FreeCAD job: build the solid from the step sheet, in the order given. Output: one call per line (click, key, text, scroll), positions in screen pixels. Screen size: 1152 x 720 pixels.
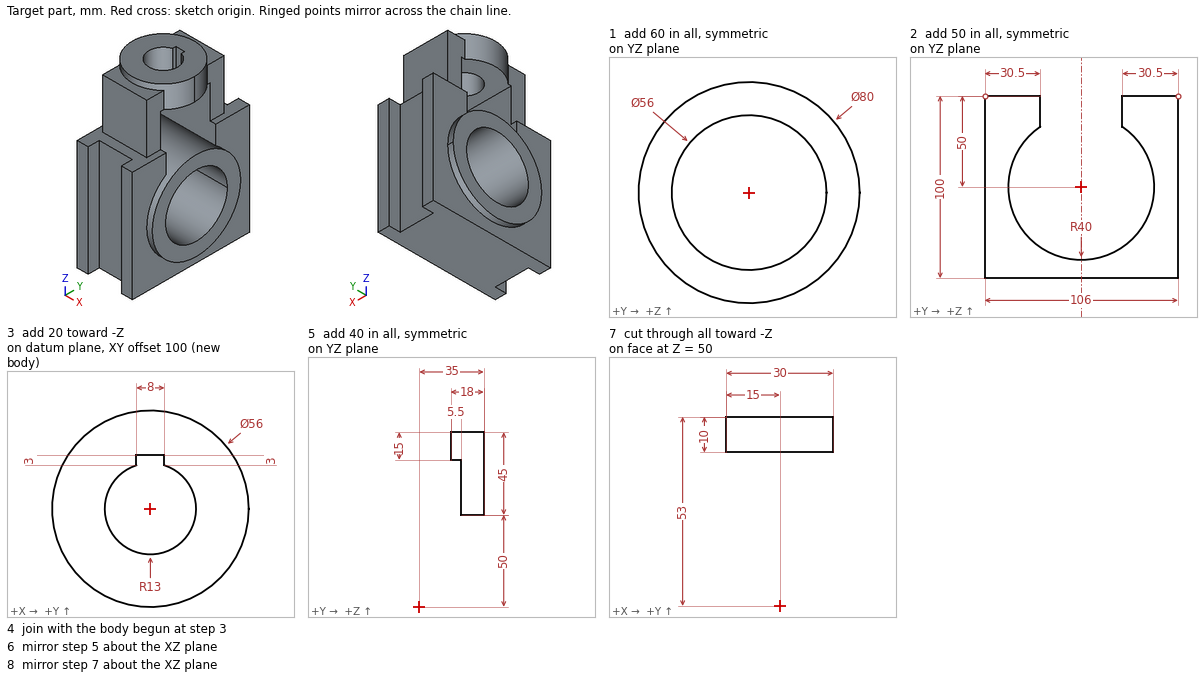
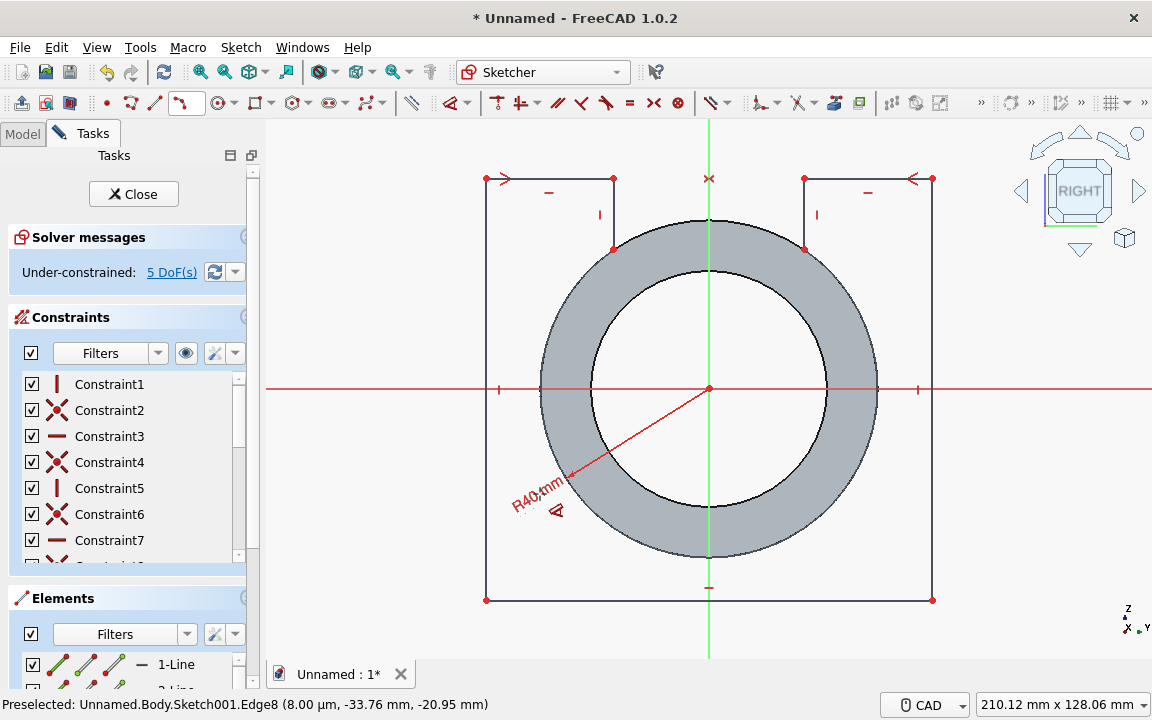
click(486, 306)
click(452, 293)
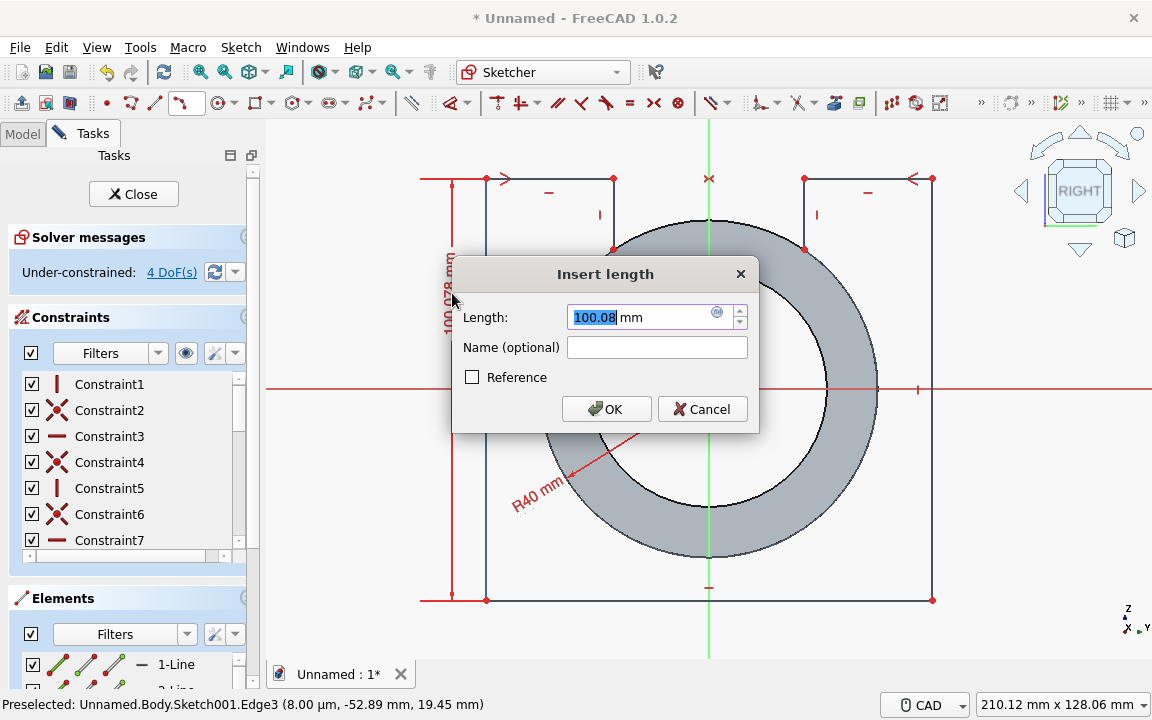
text(100)
key(Return)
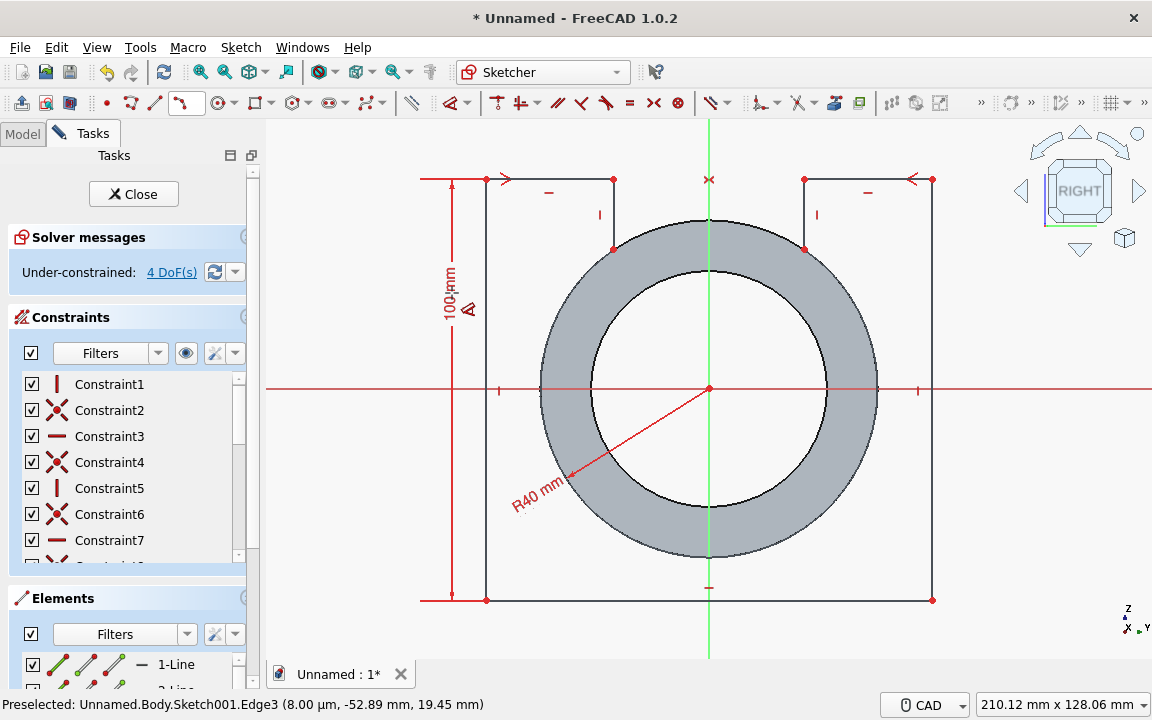
click(620, 601)
click(606, 567)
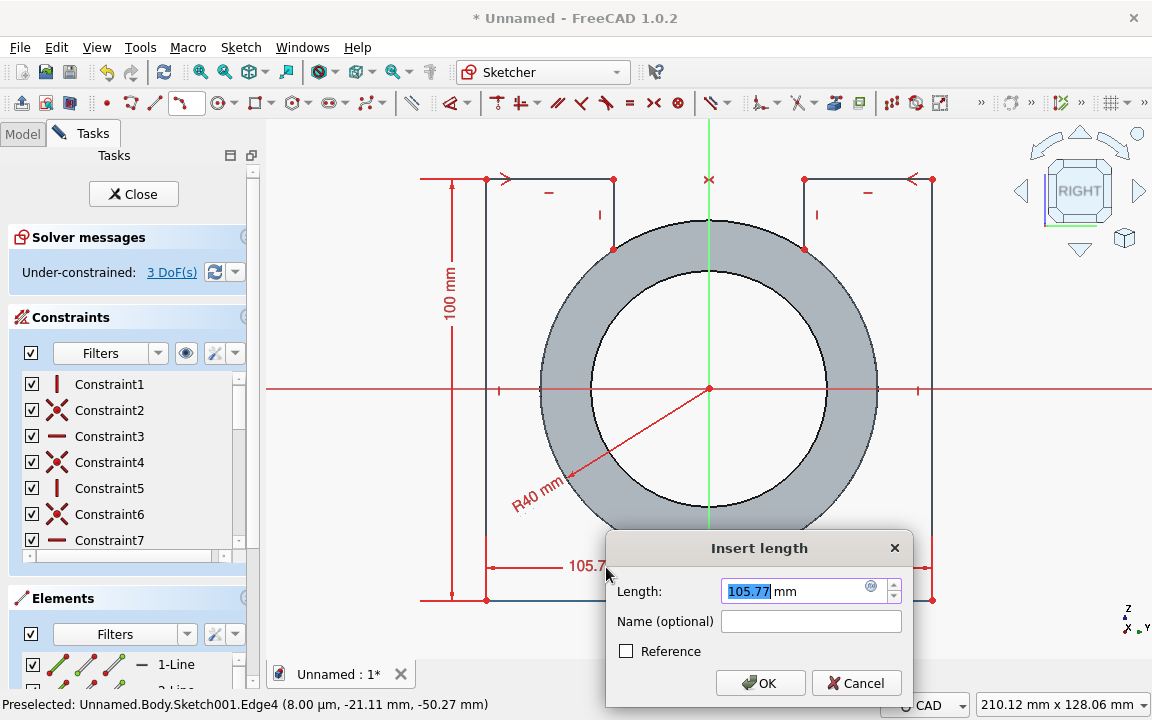
text(106)
key(Return)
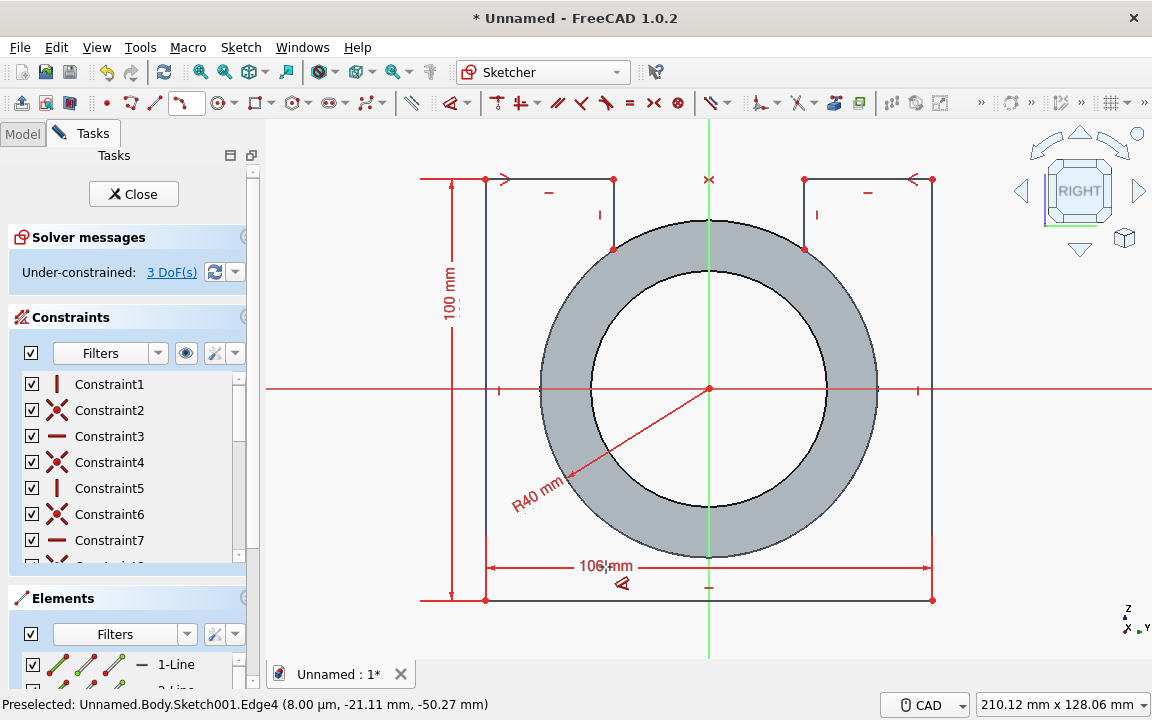
click(614, 179)
click(580, 236)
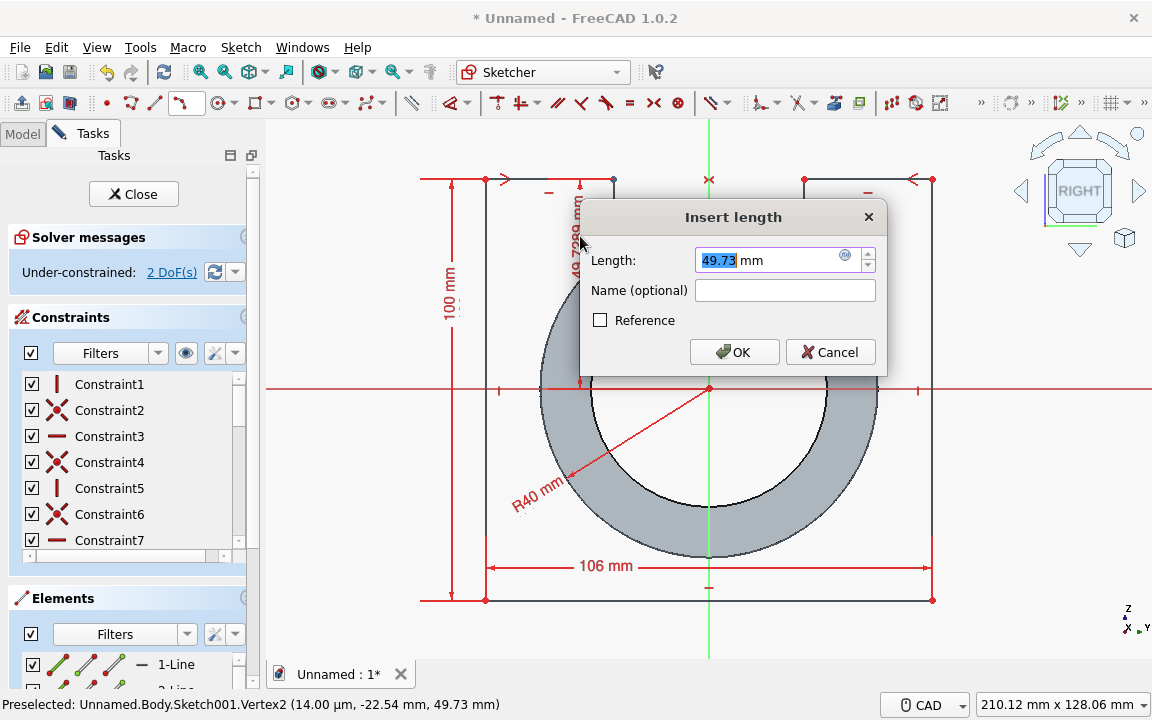
text(50)
key(Return)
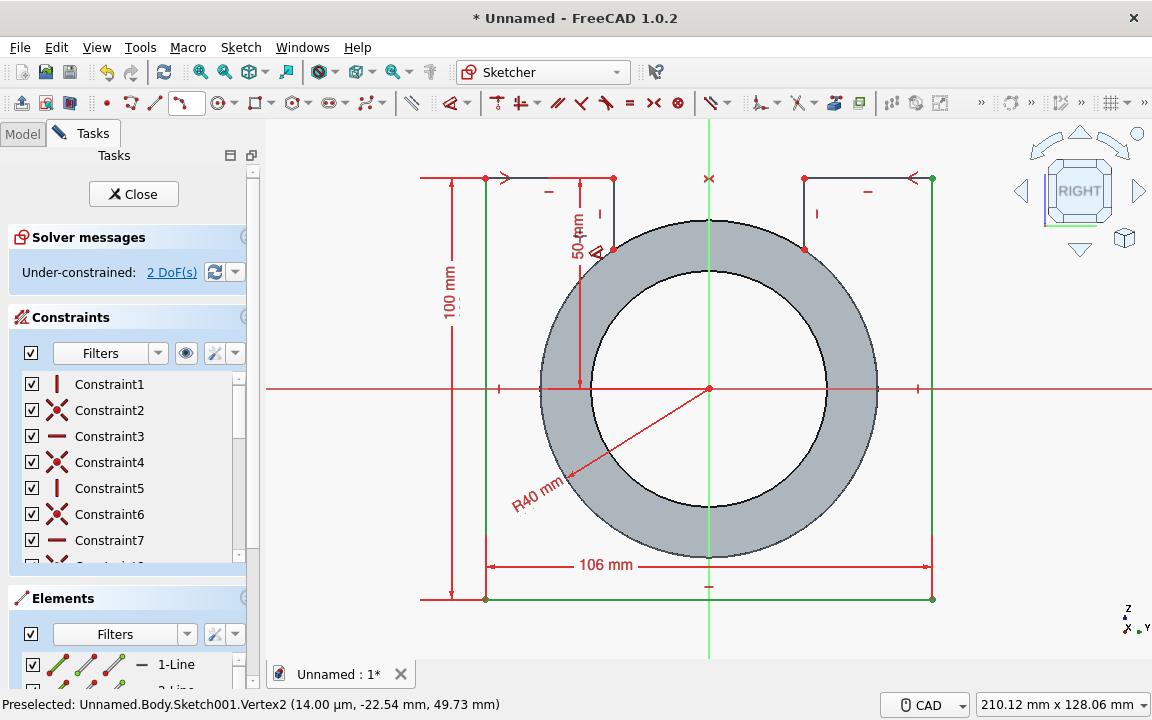
click(575, 178)
click(550, 212)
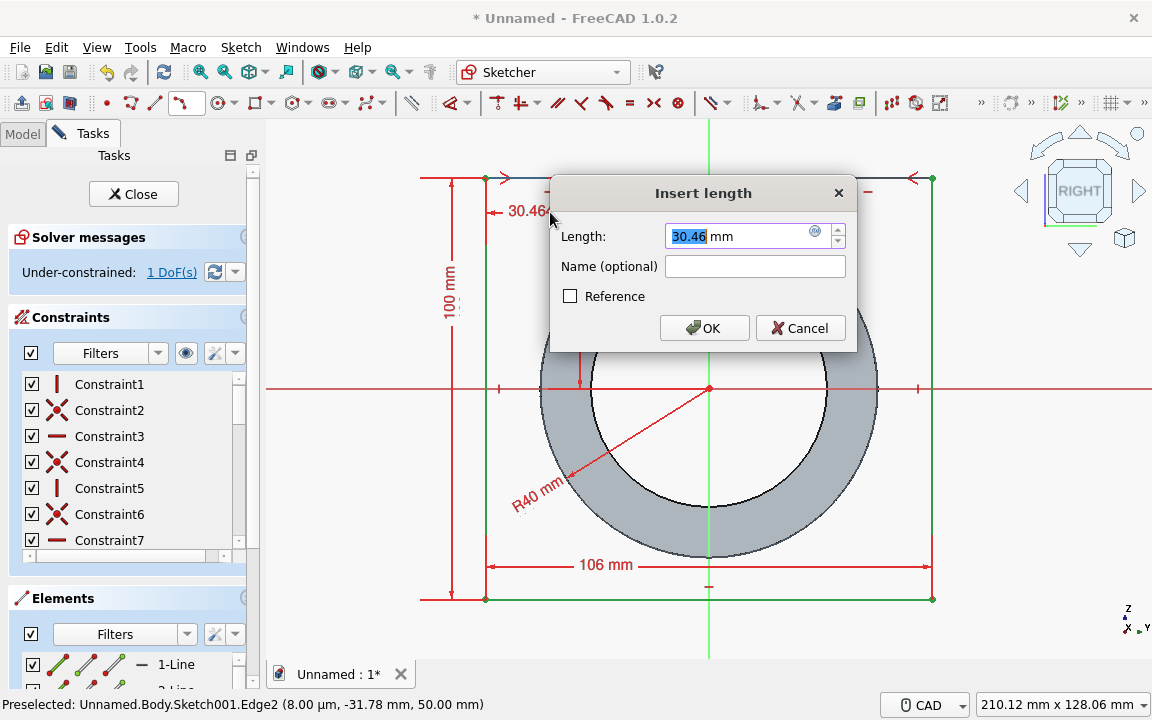
text(30.5)
key(Return)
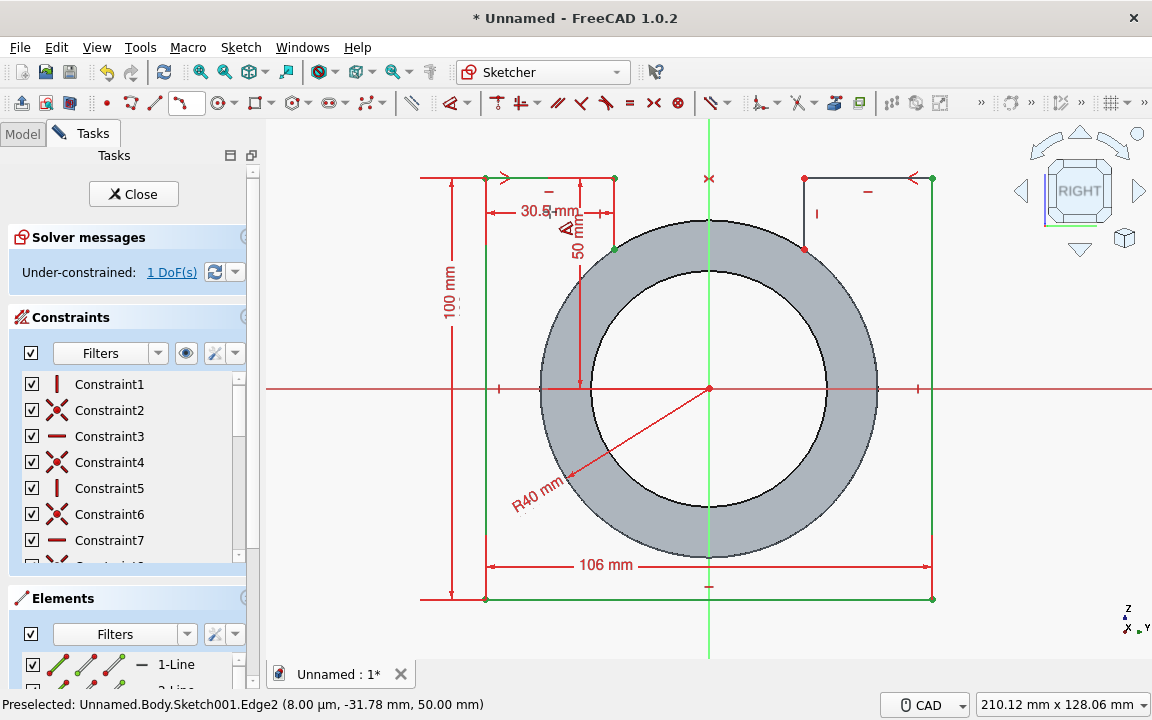
click(894, 178)
click(868, 212)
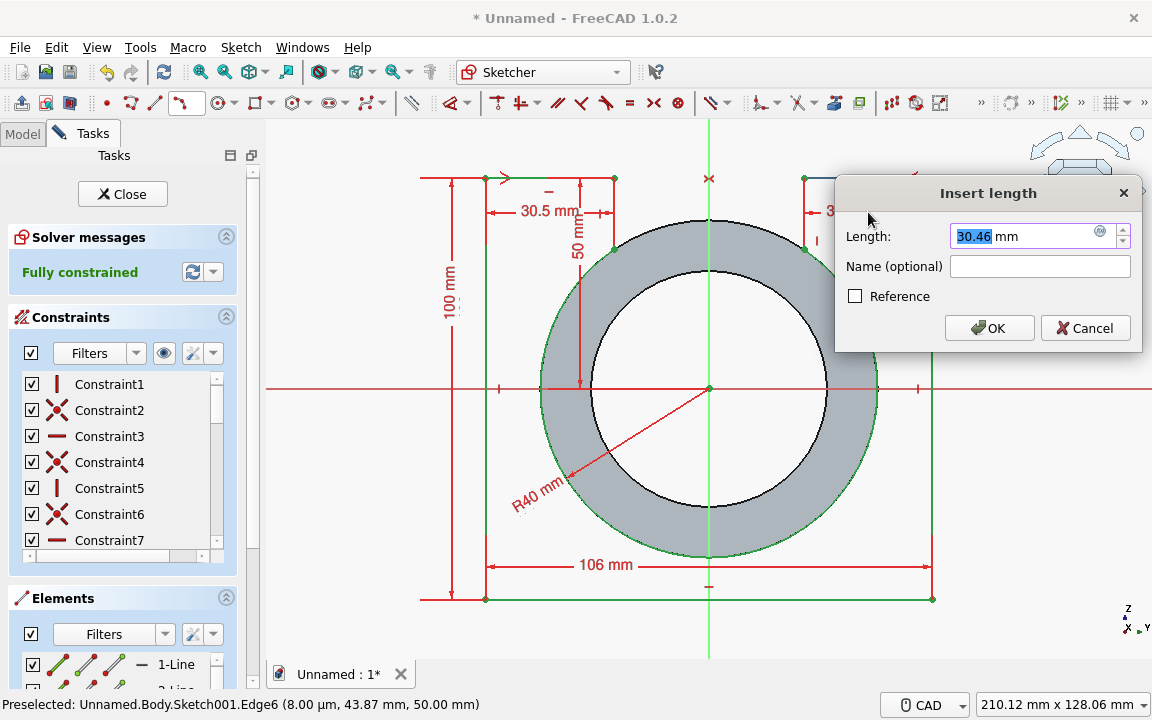
text(30.5)
key(Return)
key(Escape)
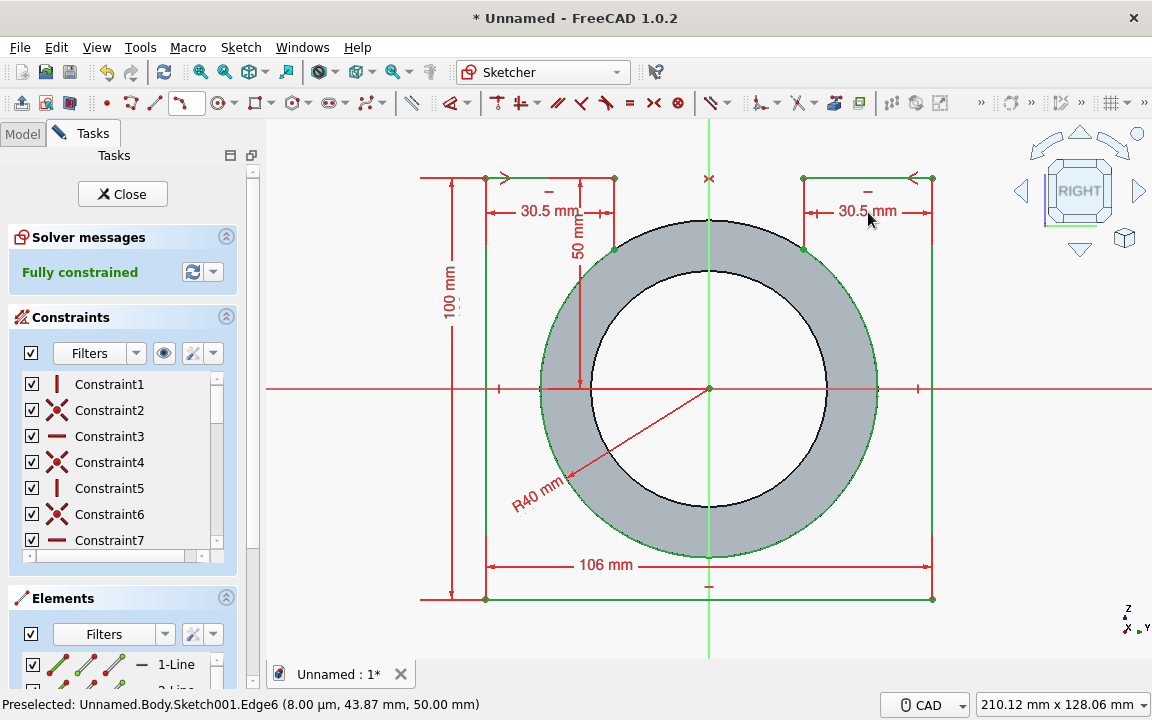
click(123, 194)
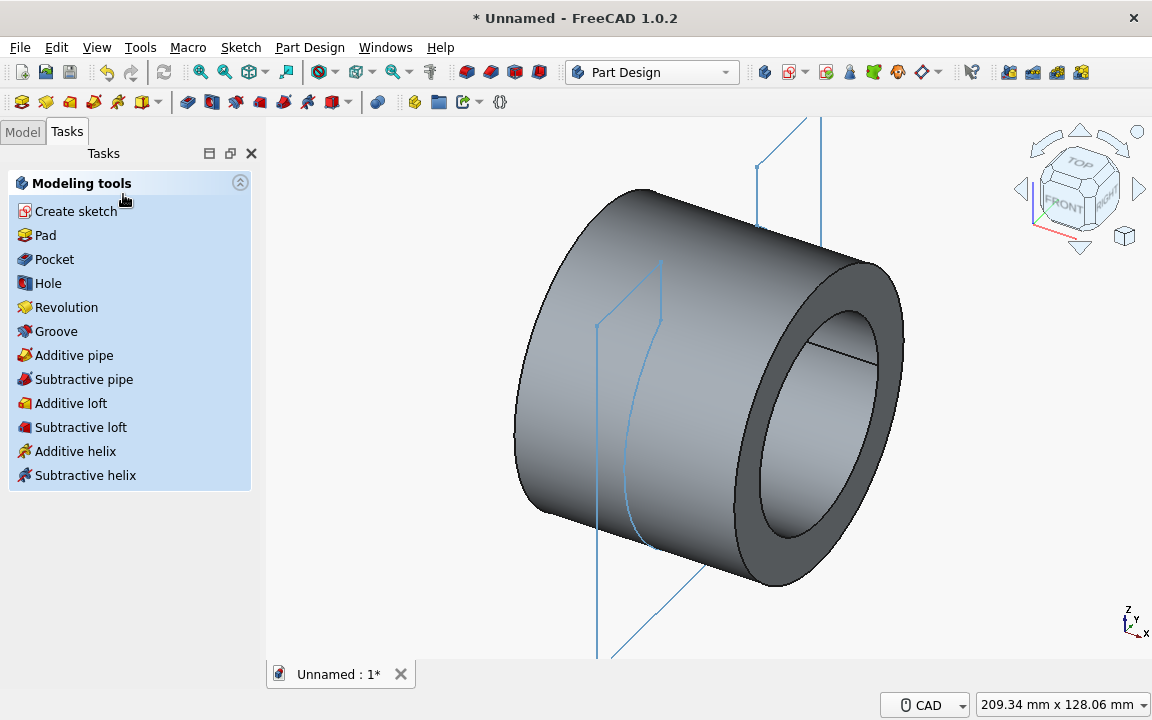
click(22, 102)